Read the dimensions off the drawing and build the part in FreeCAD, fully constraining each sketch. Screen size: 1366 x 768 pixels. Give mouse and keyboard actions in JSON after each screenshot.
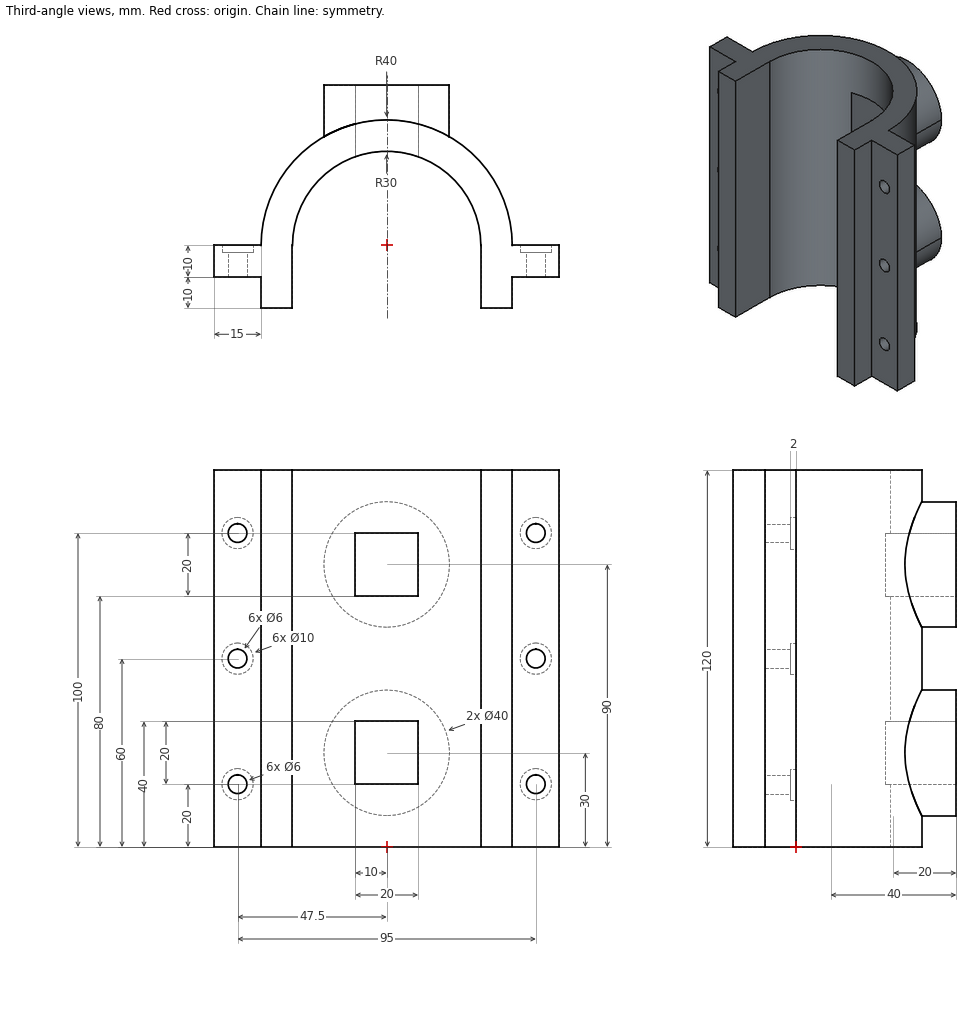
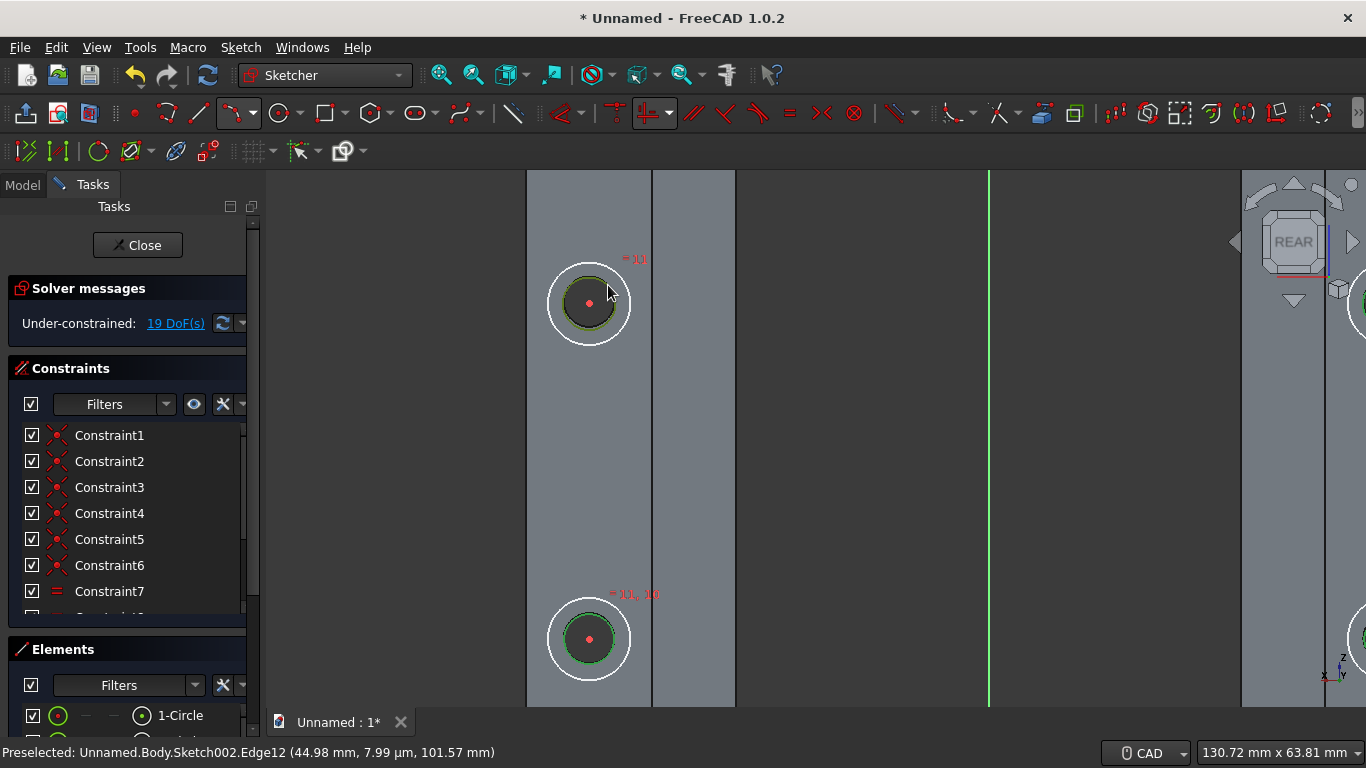
{"action": "left_click", "coordinate": [790, 114]}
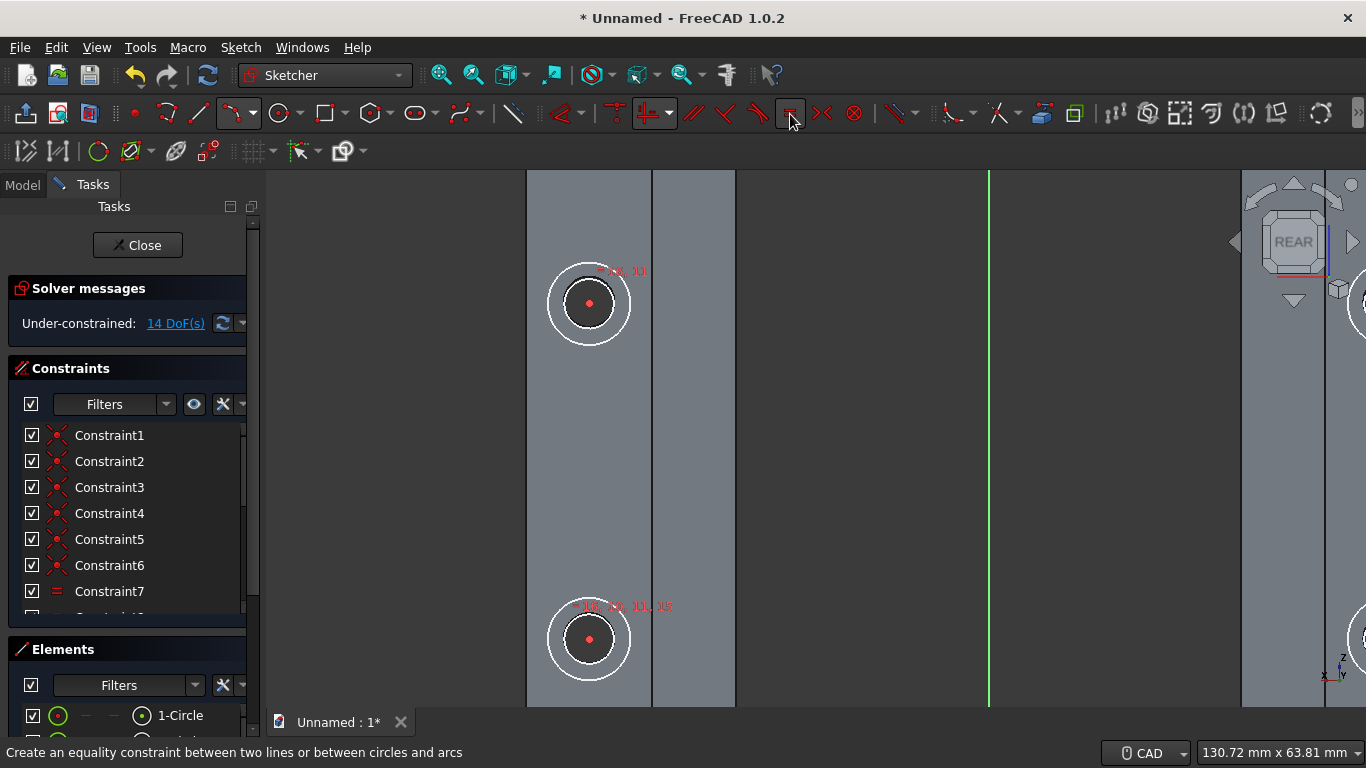
{"action": "scroll", "coordinate": [607, 286], "scroll_direction": "down", "scroll_amount": 5}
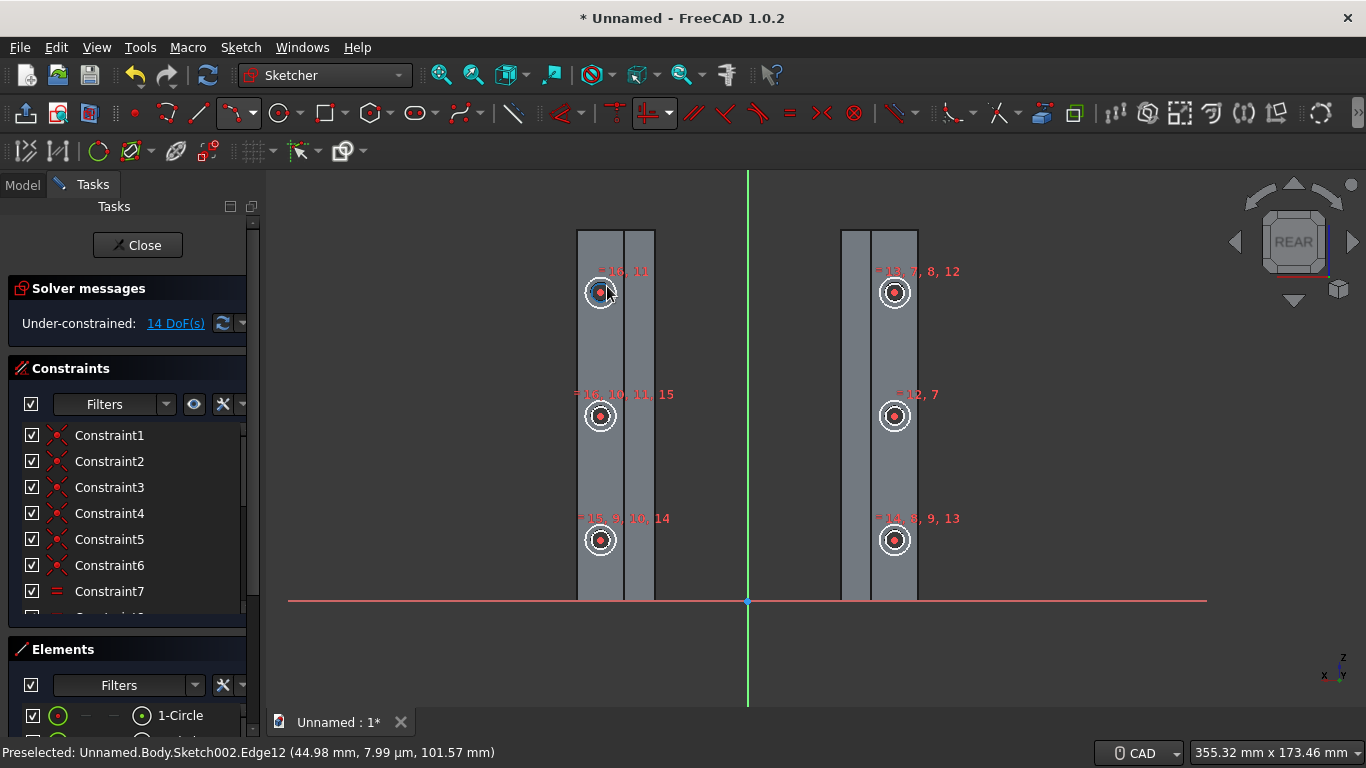
{"action": "left_click", "coordinate": [895, 416]}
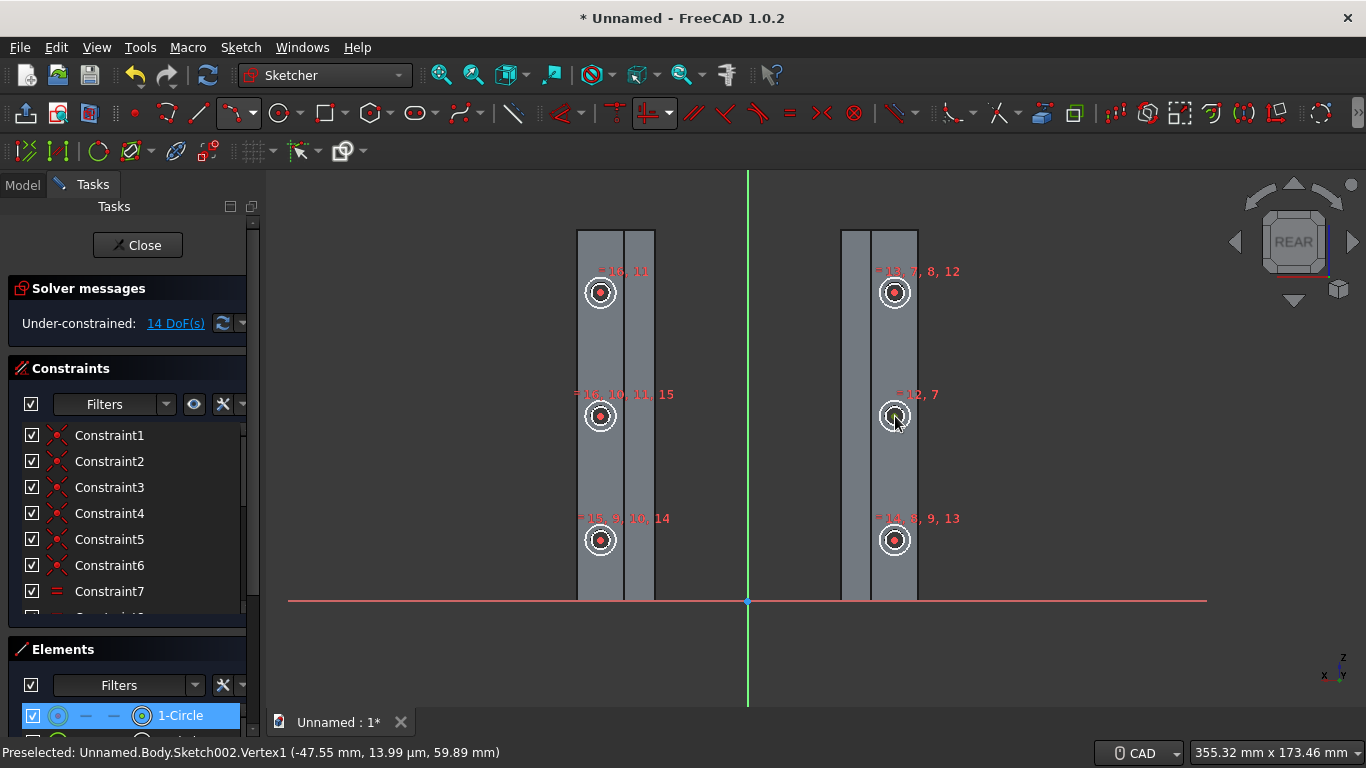
{"action": "left_click", "coordinate": [895, 293]}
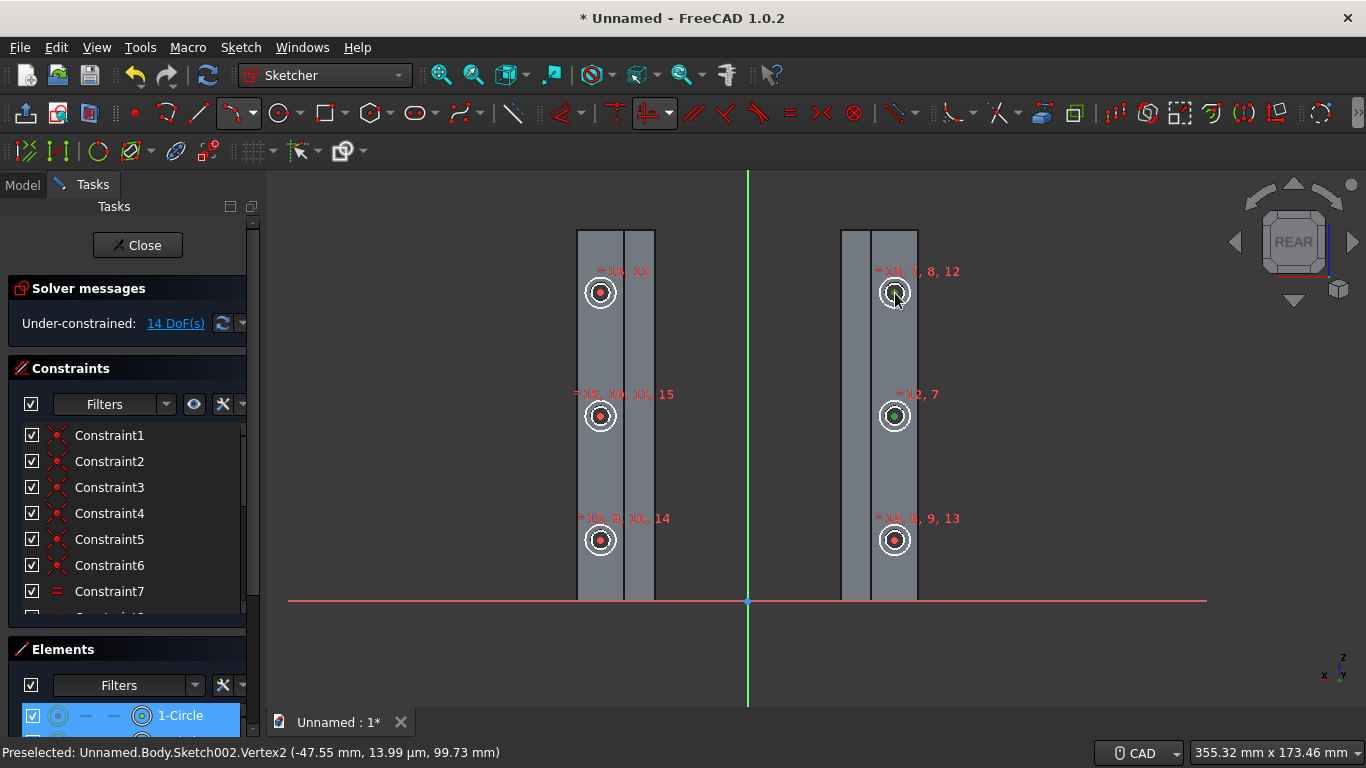
{"action": "left_click", "coordinate": [672, 114]}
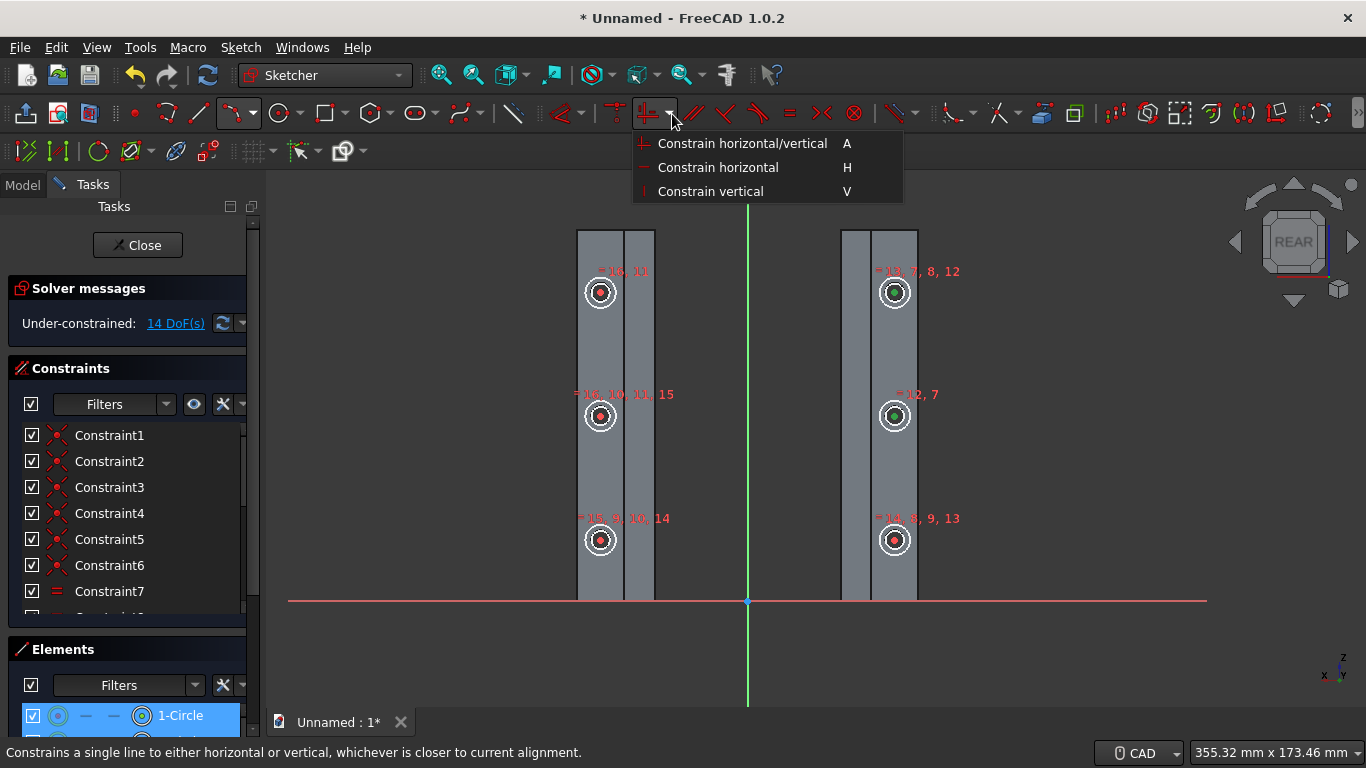
{"action": "left_click", "coordinate": [768, 191]}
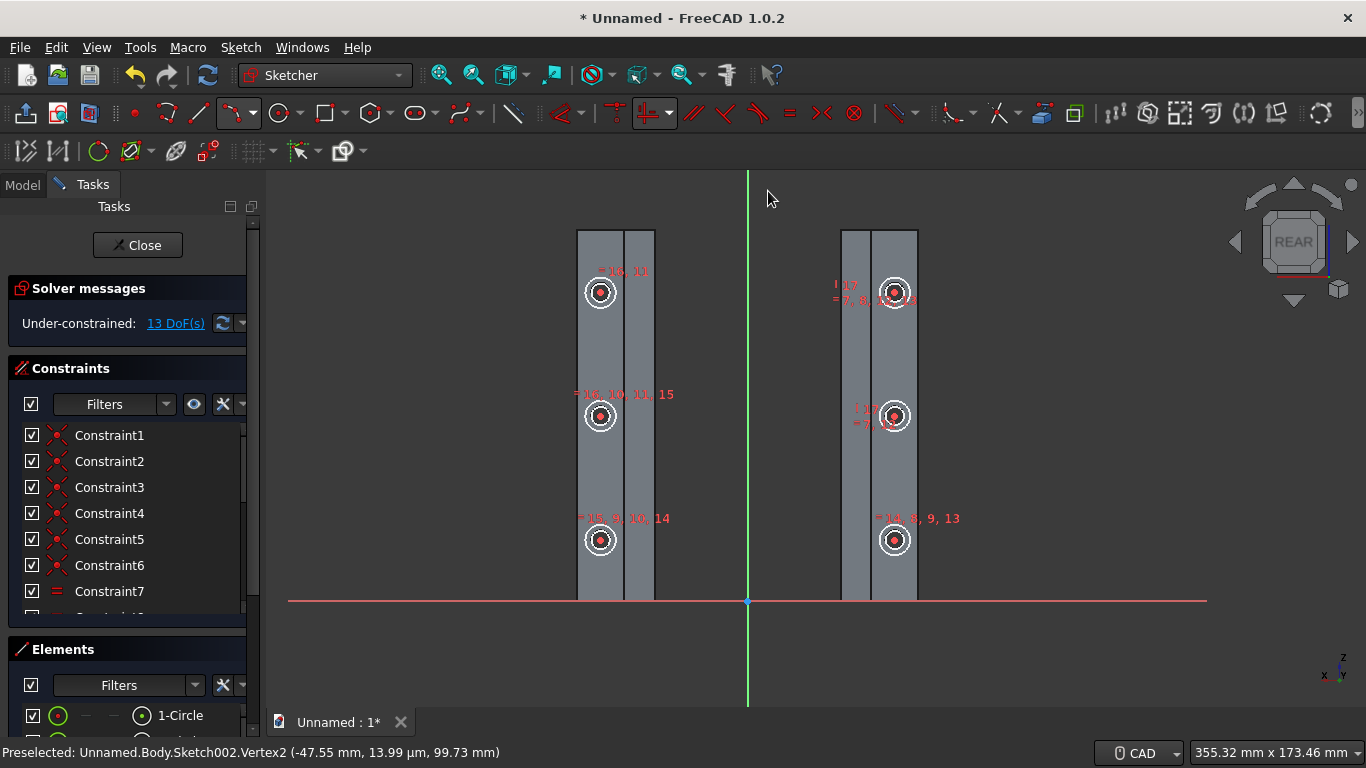
{"action": "left_click", "coordinate": [895, 416]}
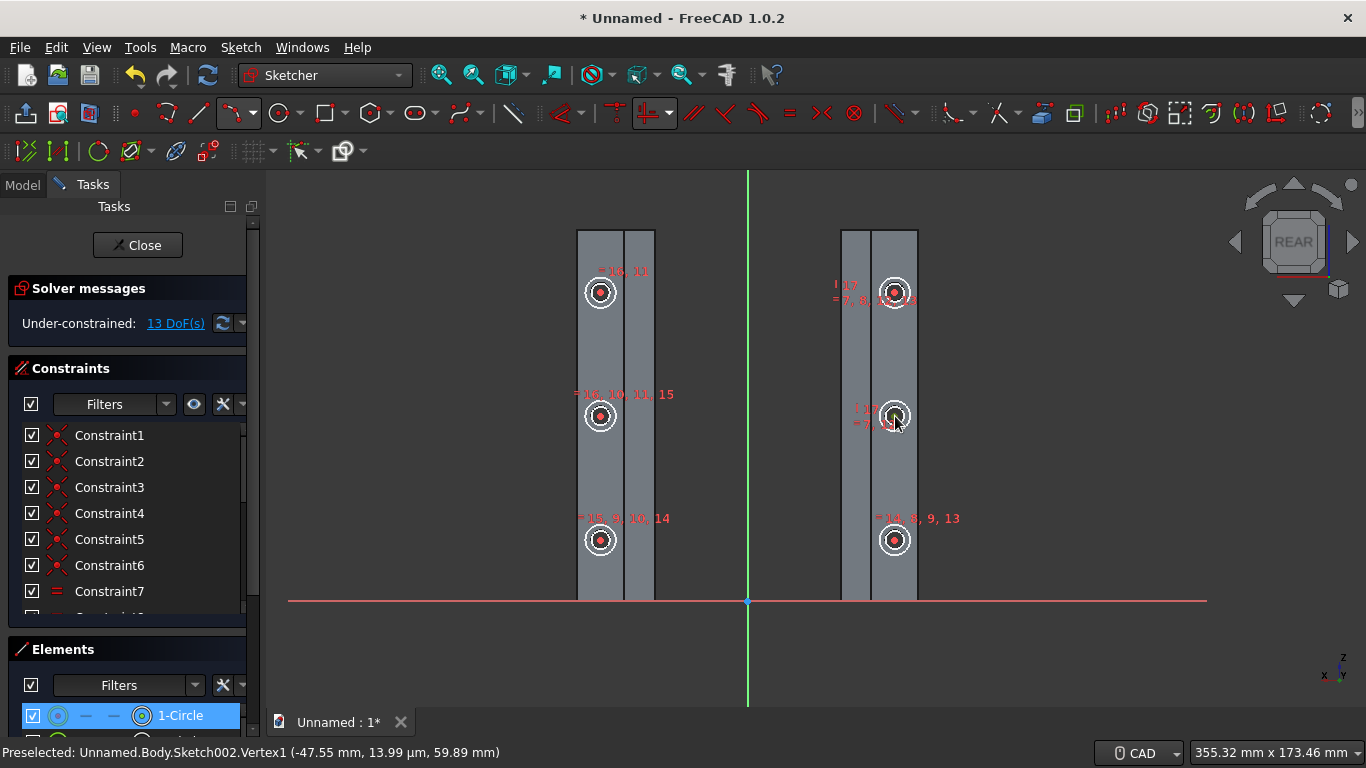
{"action": "left_click", "coordinate": [895, 540]}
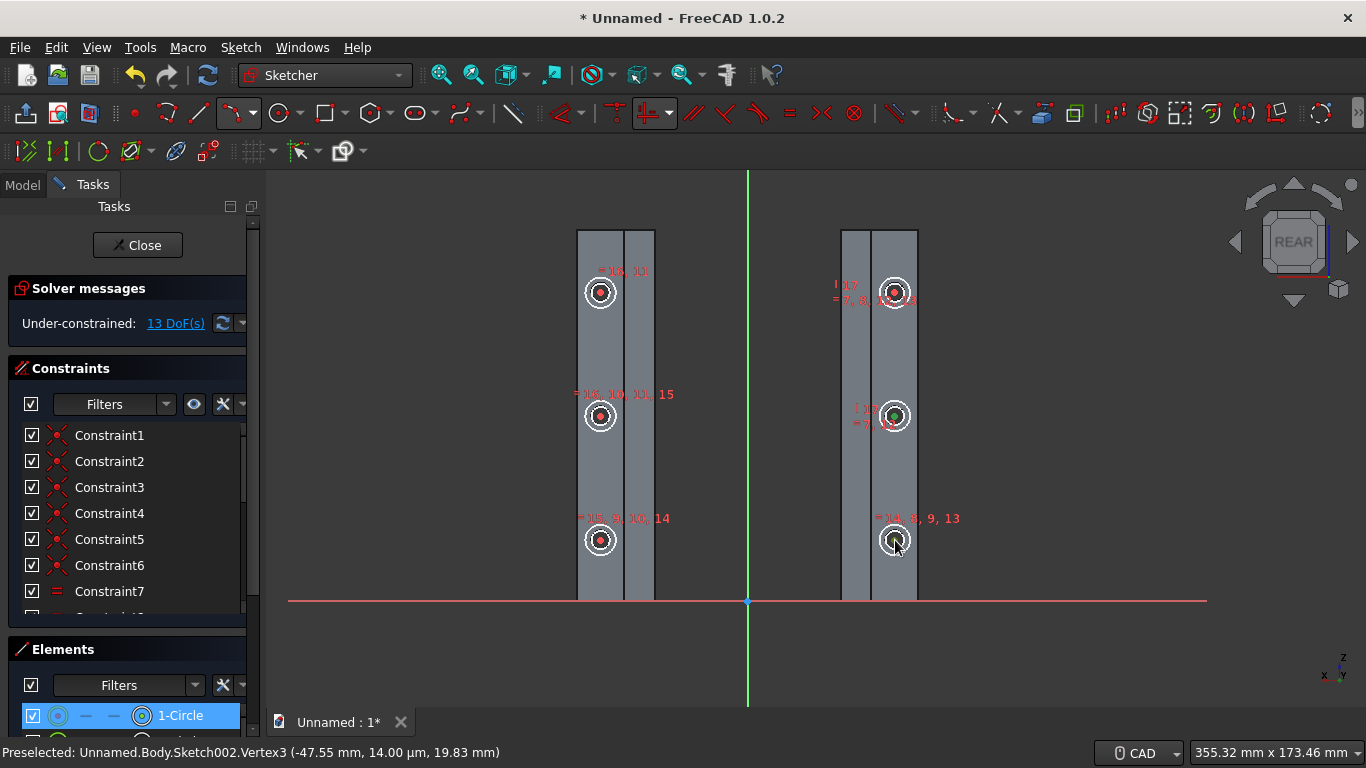
{"action": "left_click", "coordinate": [672, 114]}